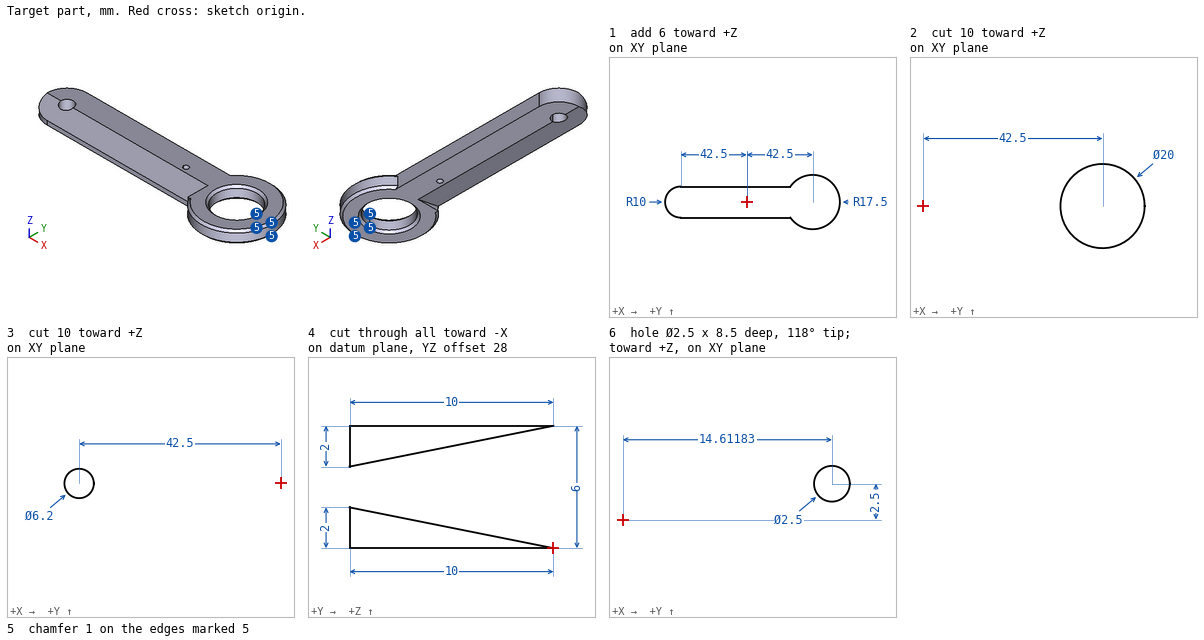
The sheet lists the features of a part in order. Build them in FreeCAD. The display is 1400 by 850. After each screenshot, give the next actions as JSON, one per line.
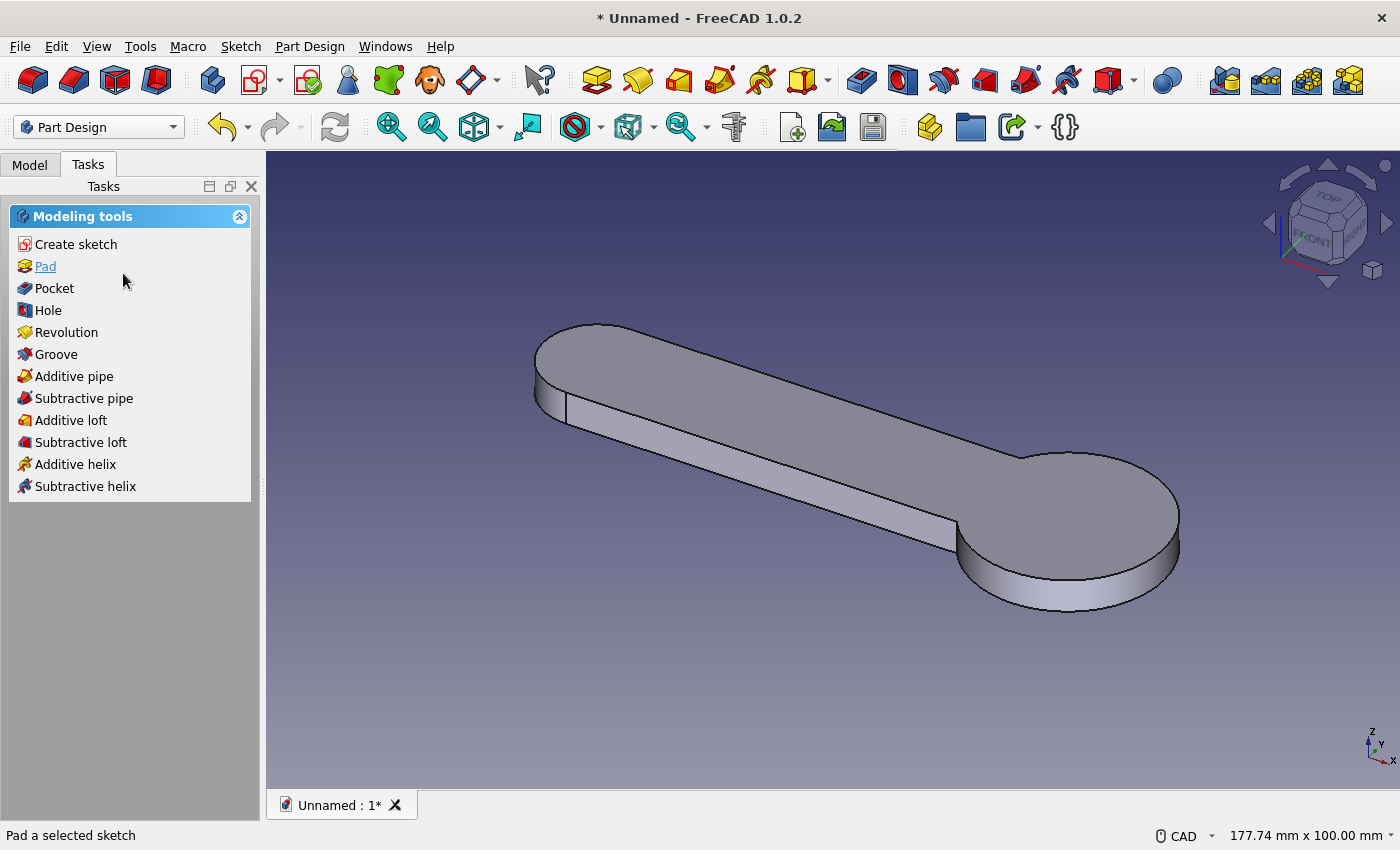
{"action": "left_click", "coordinate": [862, 80]}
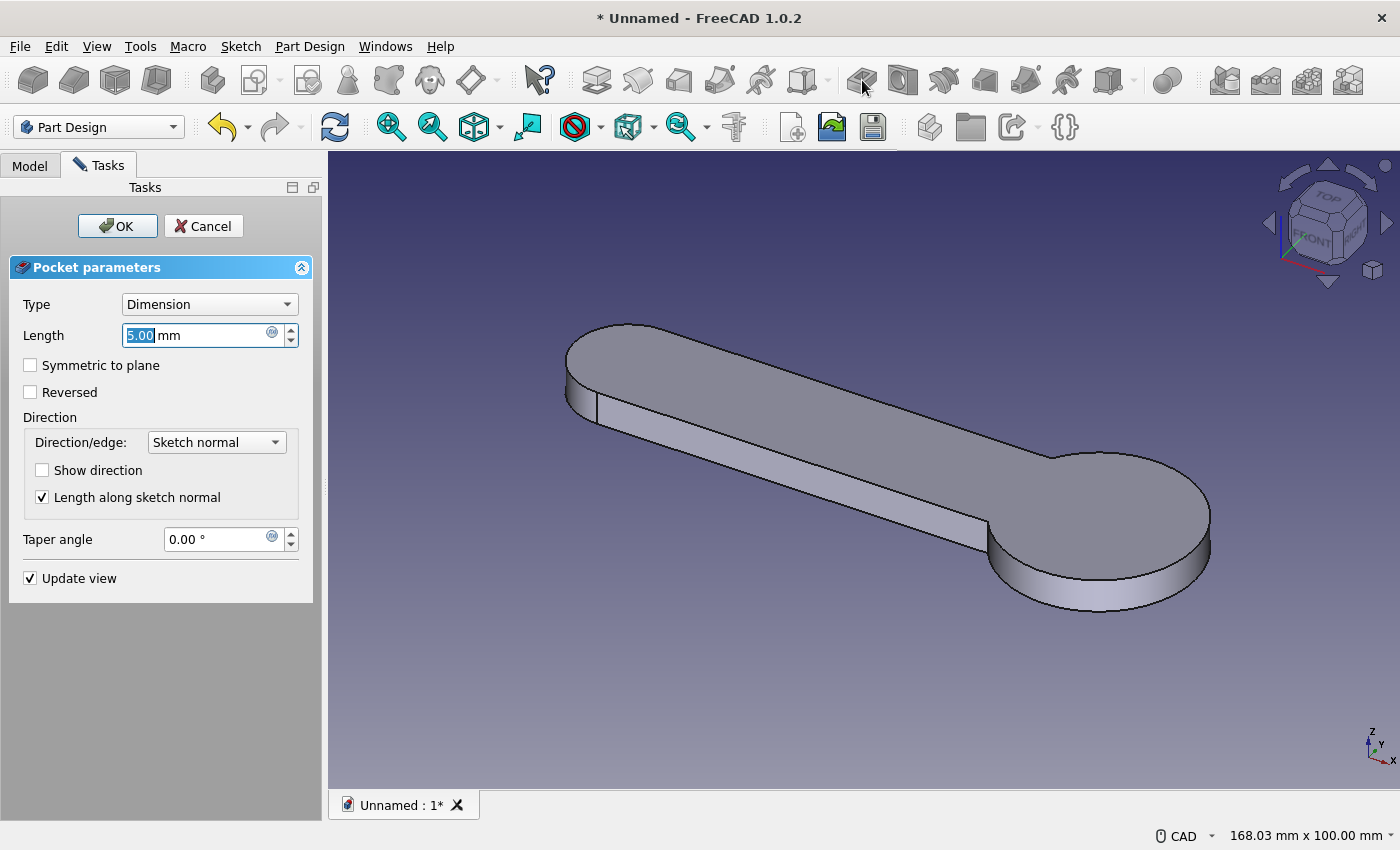
{"action": "type", "text": "10"}
{"action": "key", "text": "Tab"}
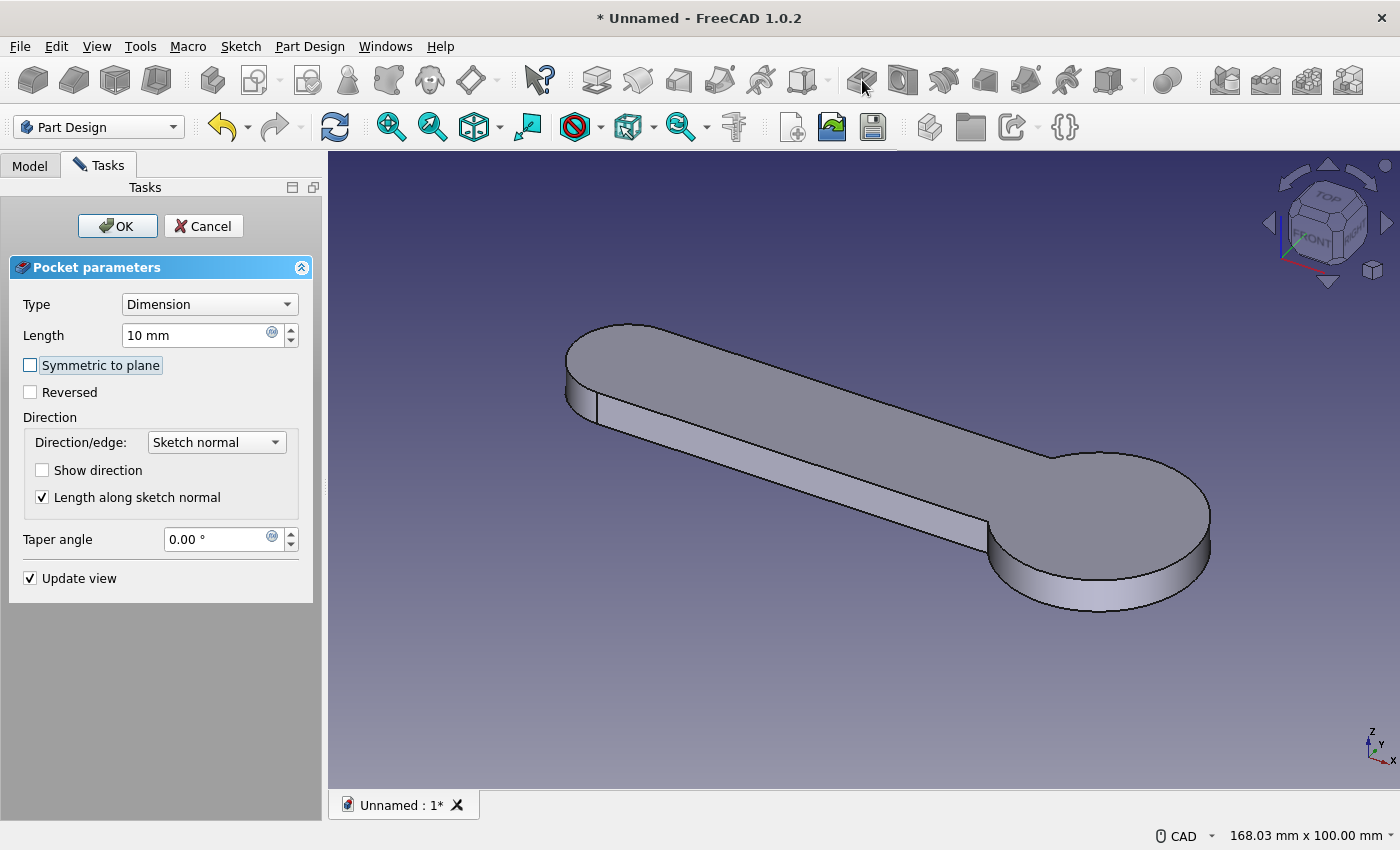
{"action": "left_click", "coordinate": [31, 392]}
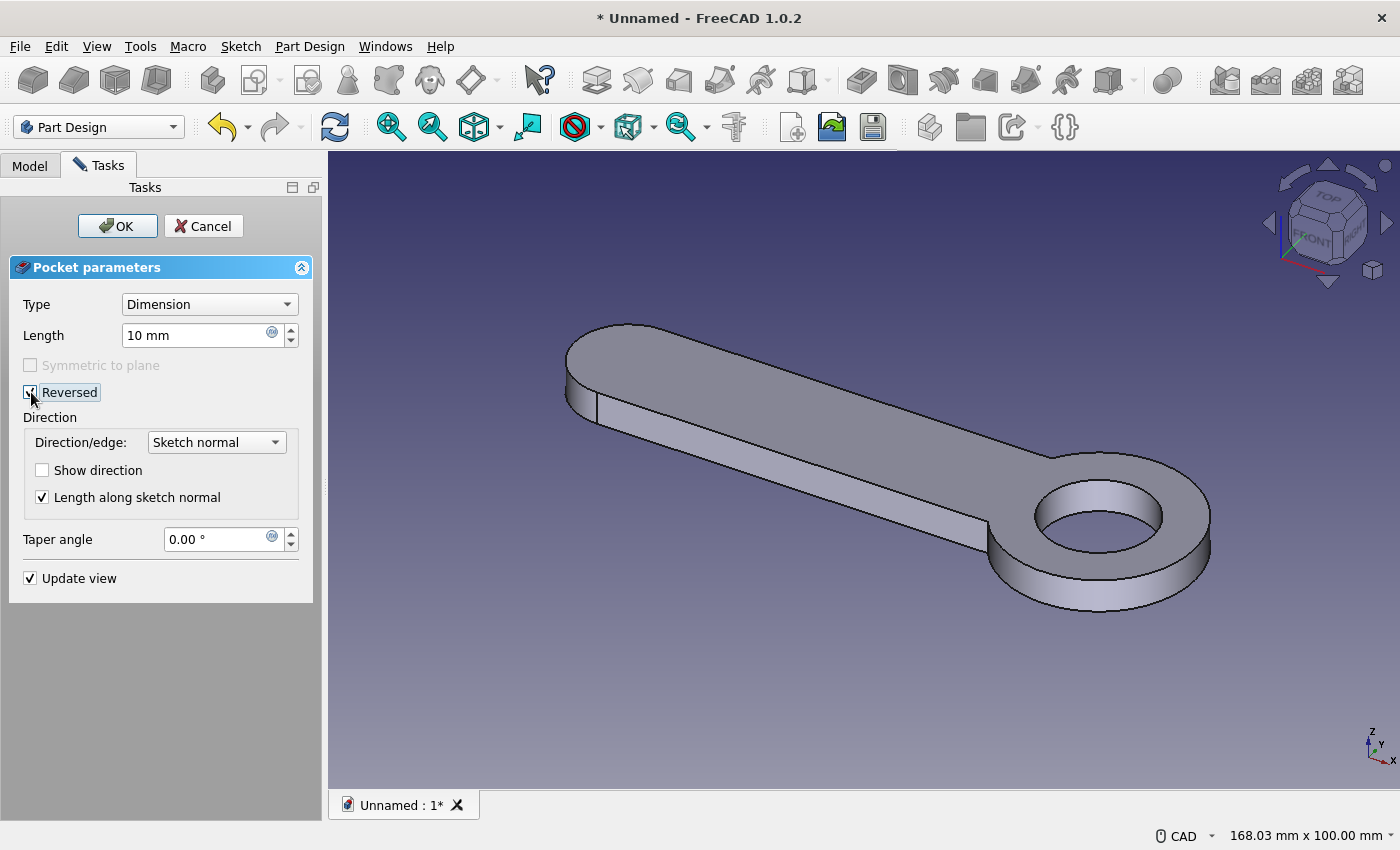
{"action": "left_click", "coordinate": [118, 226]}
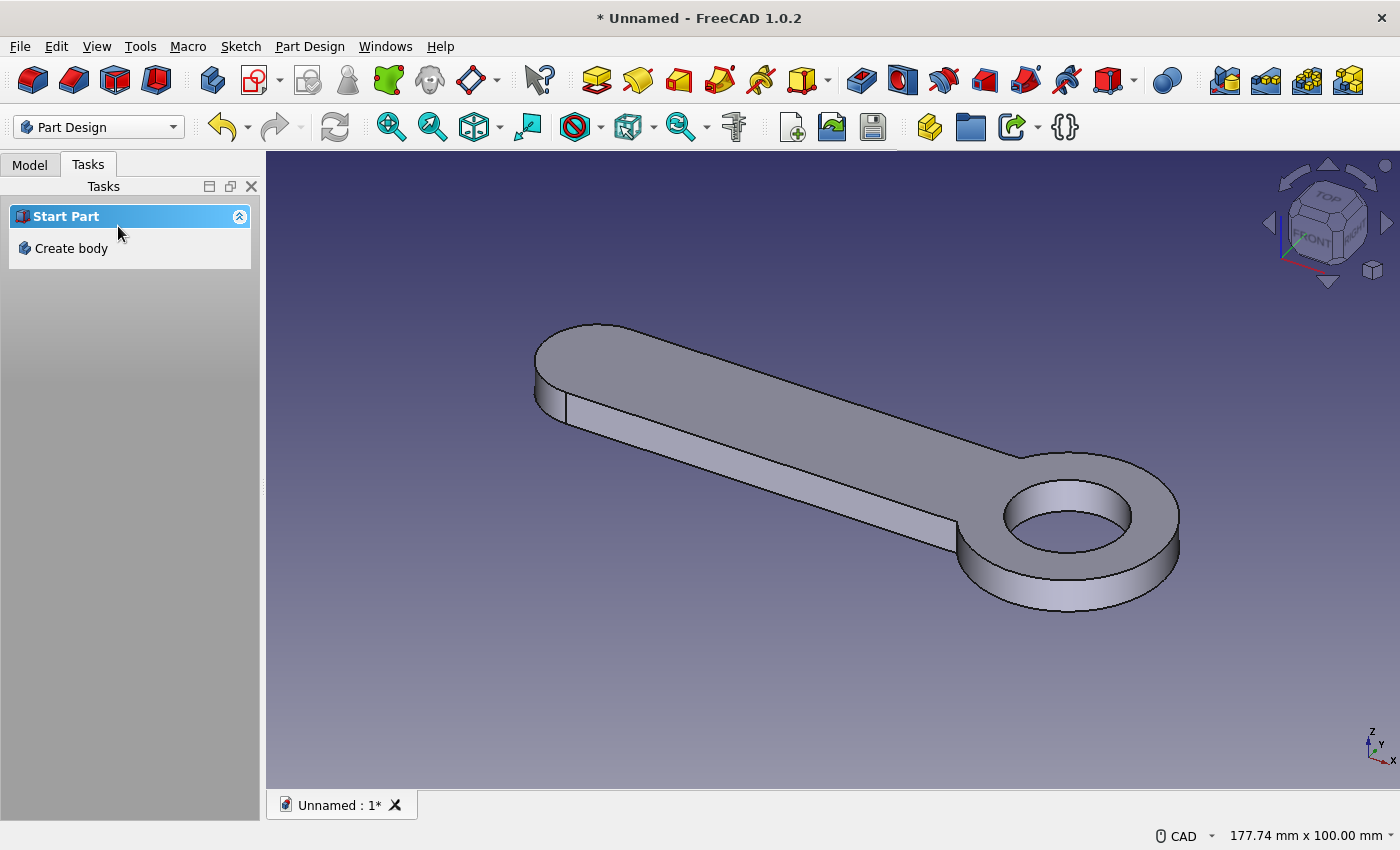
{"action": "left_click", "coordinate": [254, 80]}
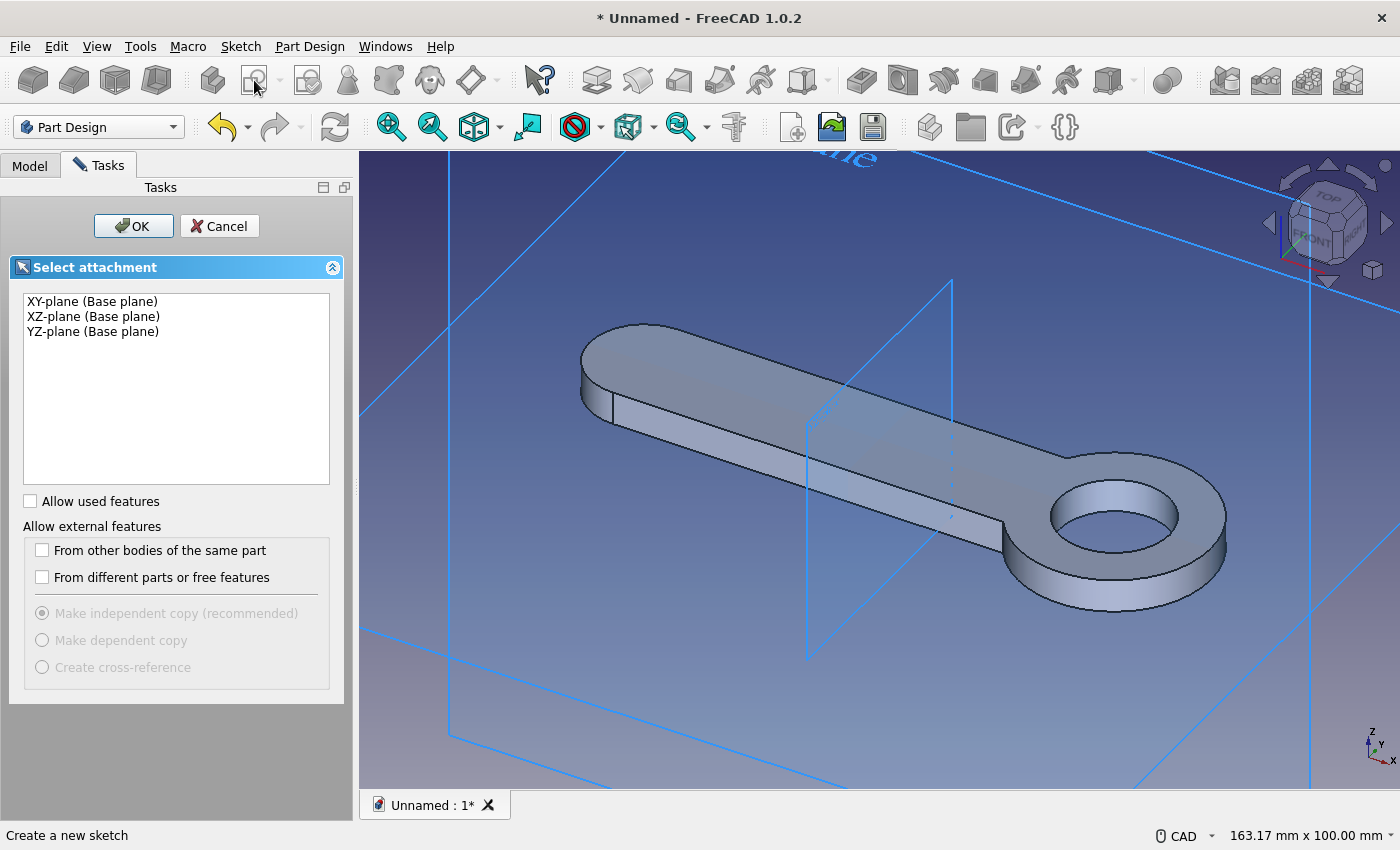
{"action": "left_click", "coordinate": [84, 302]}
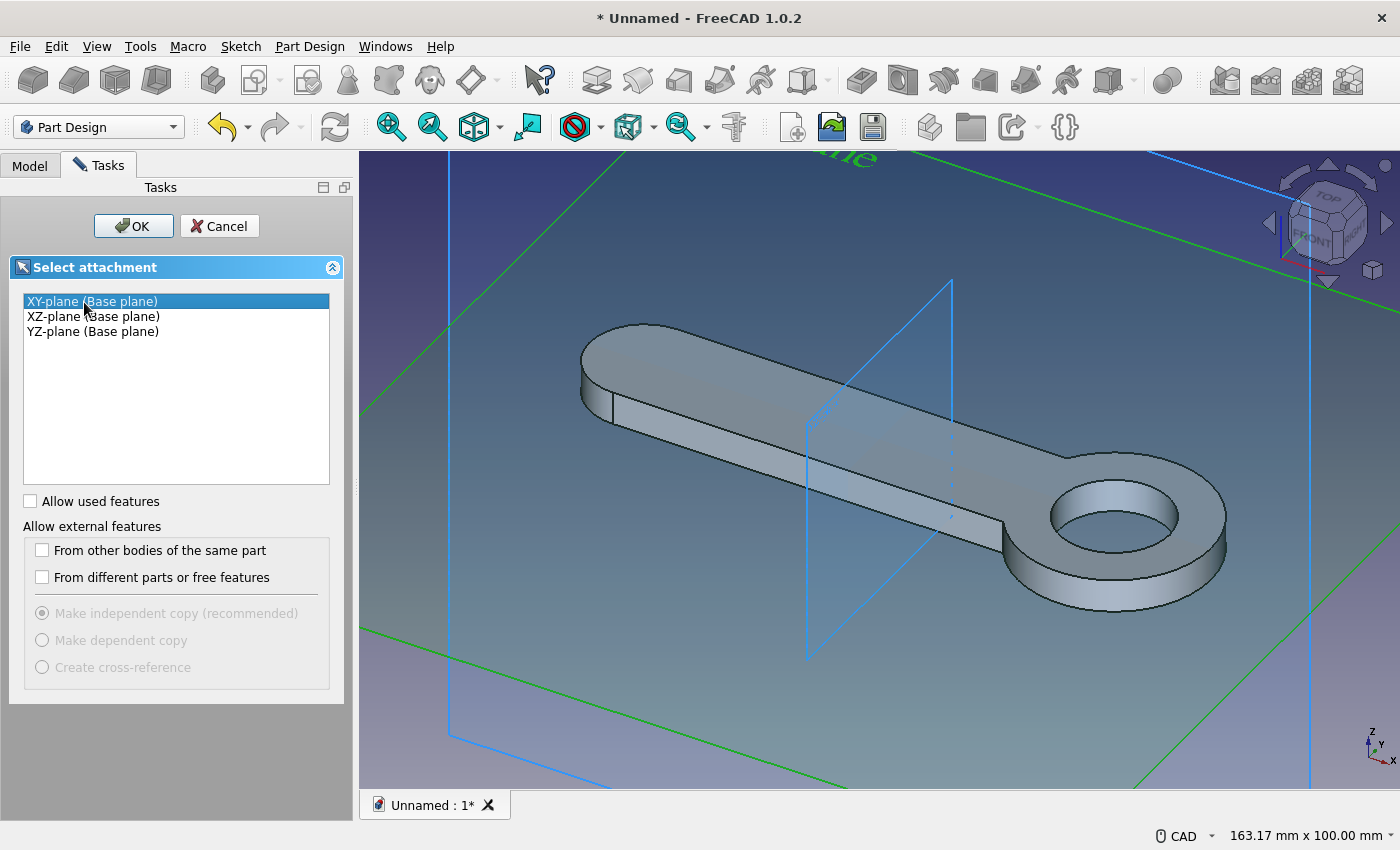
{"action": "left_click", "coordinate": [134, 226]}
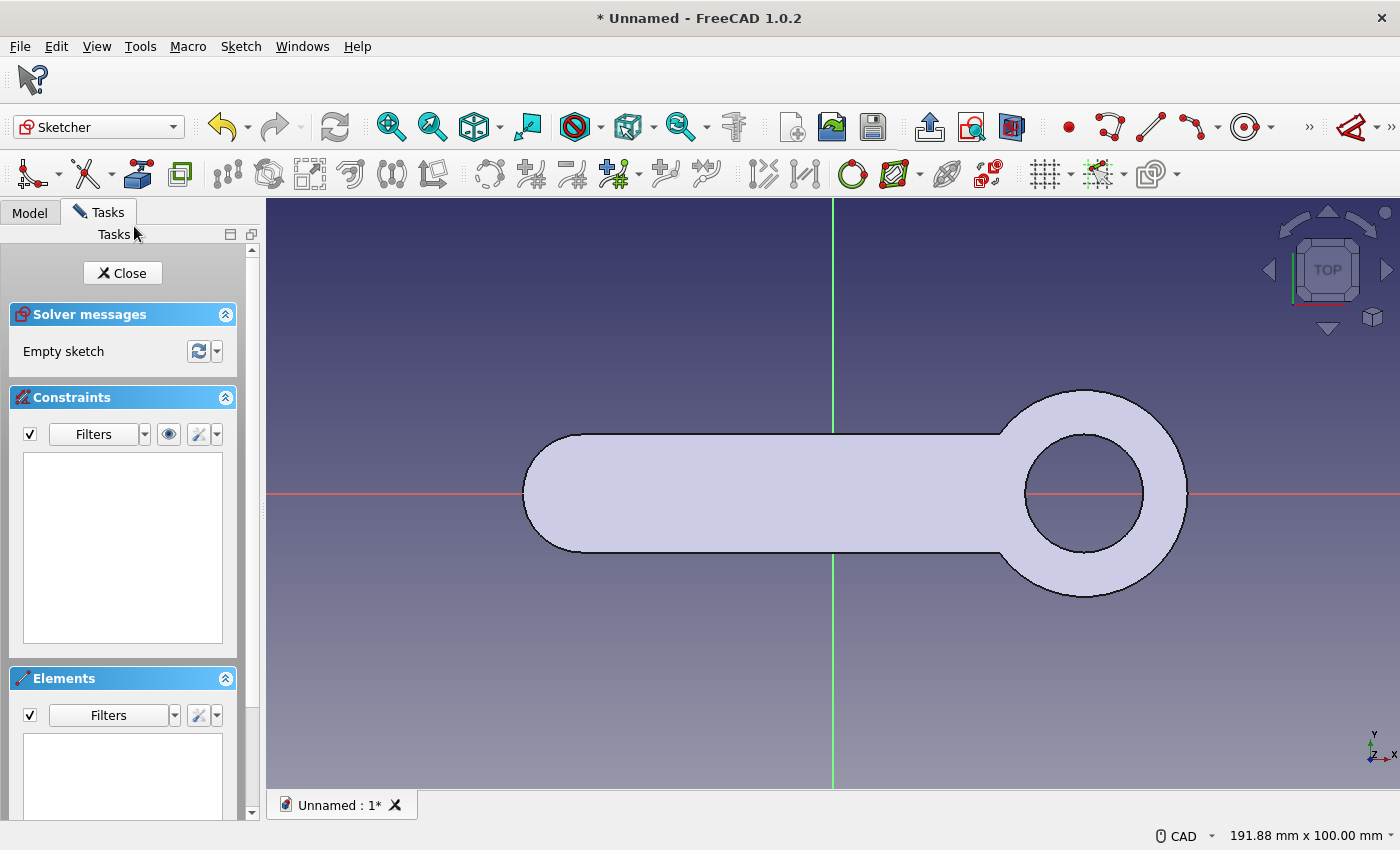
{"action": "key", "text": "q s"}